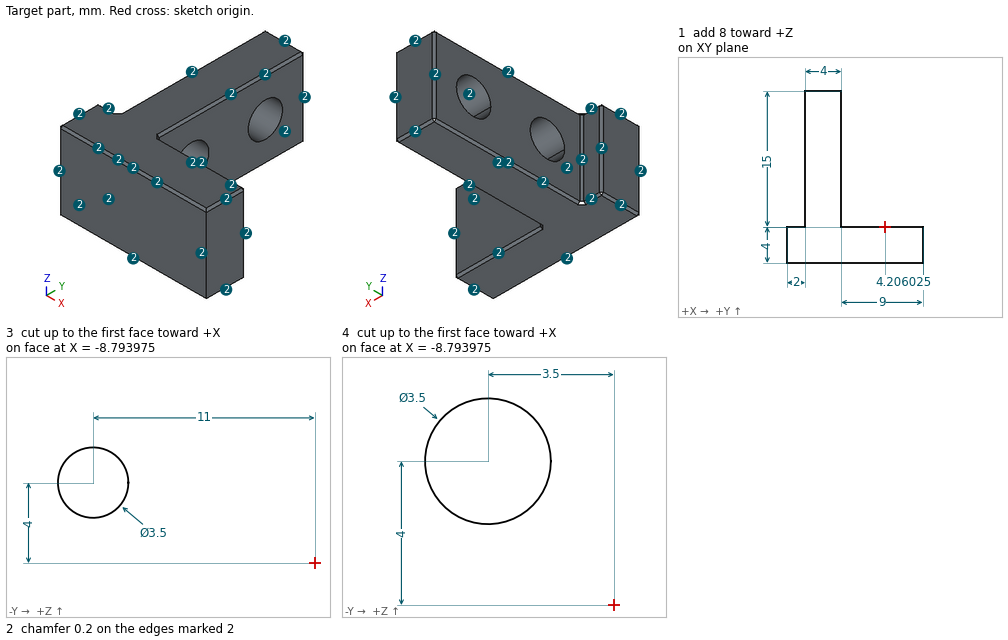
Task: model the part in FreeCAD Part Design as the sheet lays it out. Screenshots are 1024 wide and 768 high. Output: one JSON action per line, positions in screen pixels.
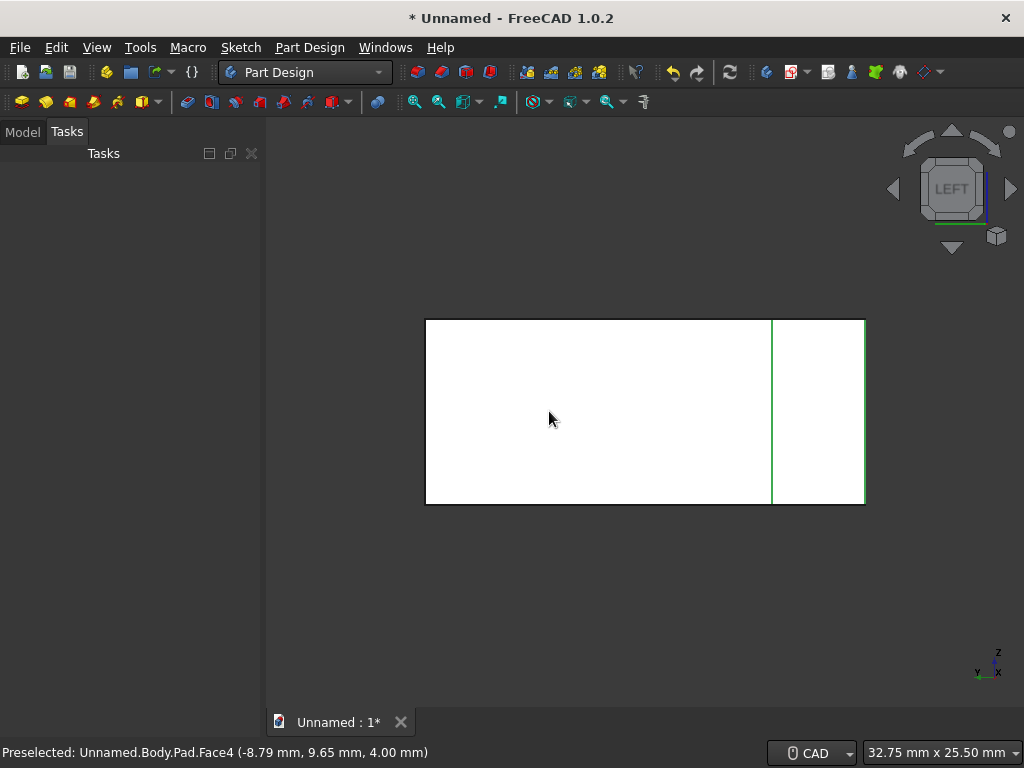
{"action": "left_click", "coordinate": [442, 72]}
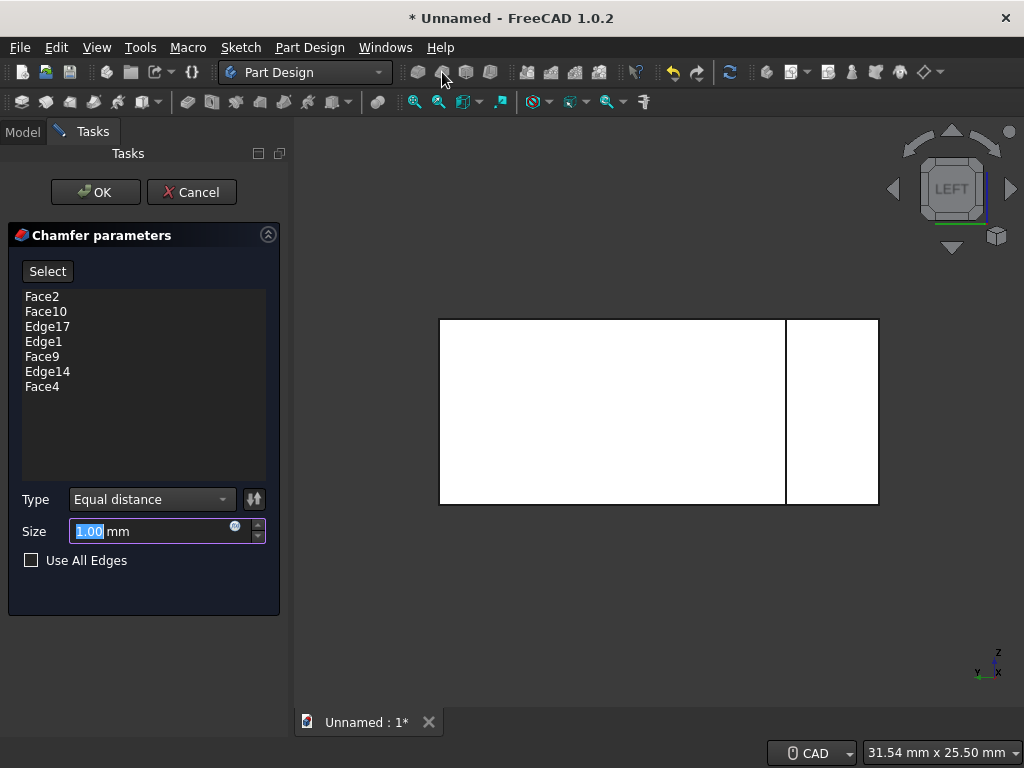
{"action": "type", "text": "0.2"}
{"action": "key", "text": "Tab"}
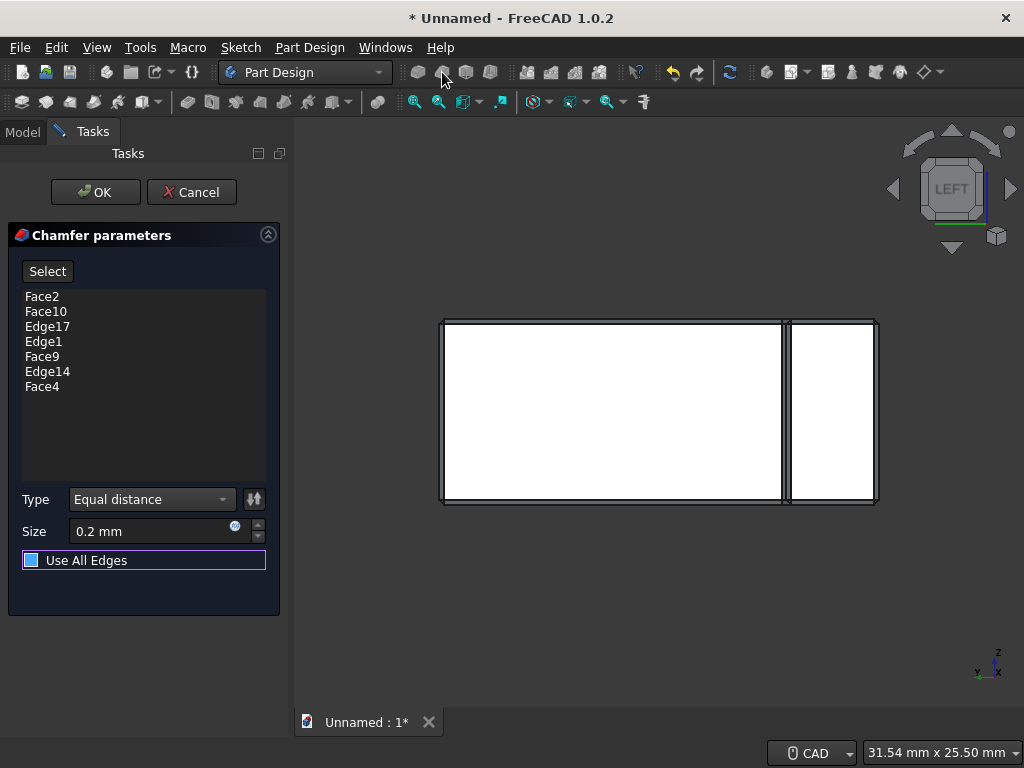
{"action": "left_click", "coordinate": [96, 192]}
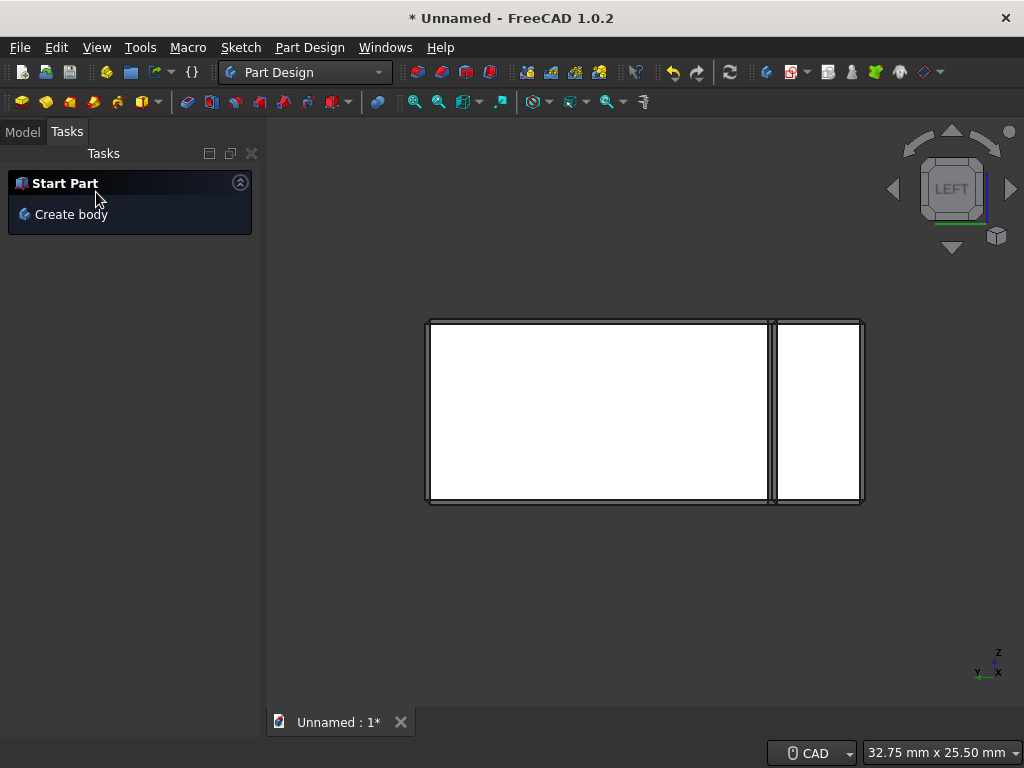
{"action": "left_click", "coordinate": [550, 411]}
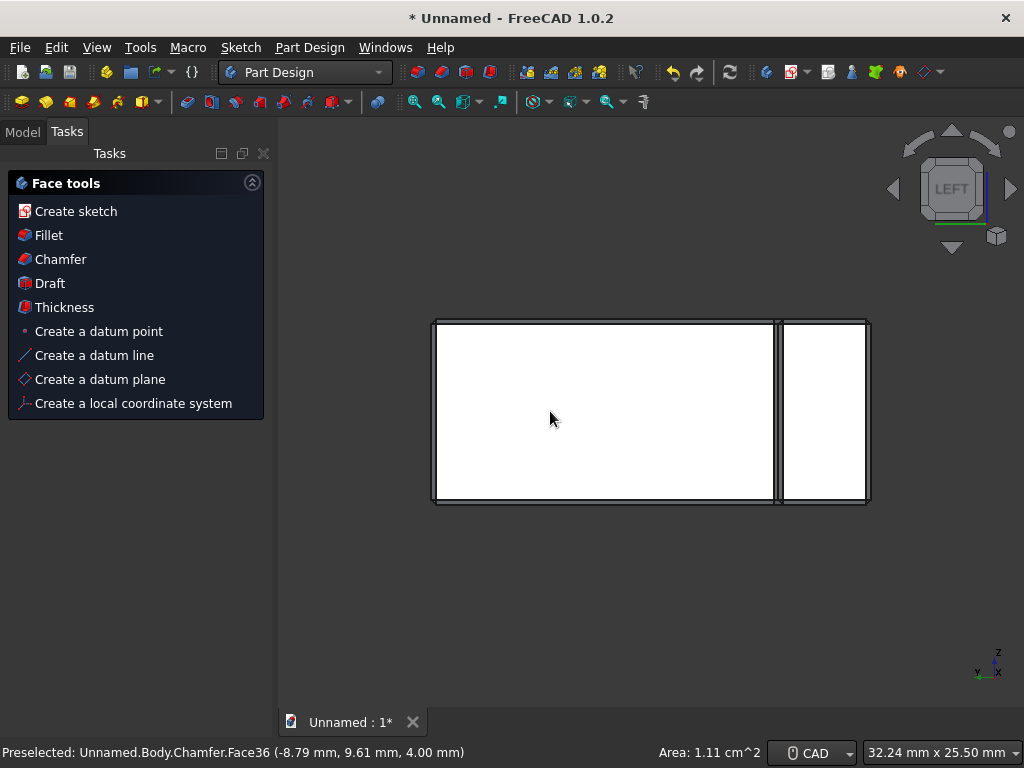
{"action": "left_click", "coordinate": [792, 72]}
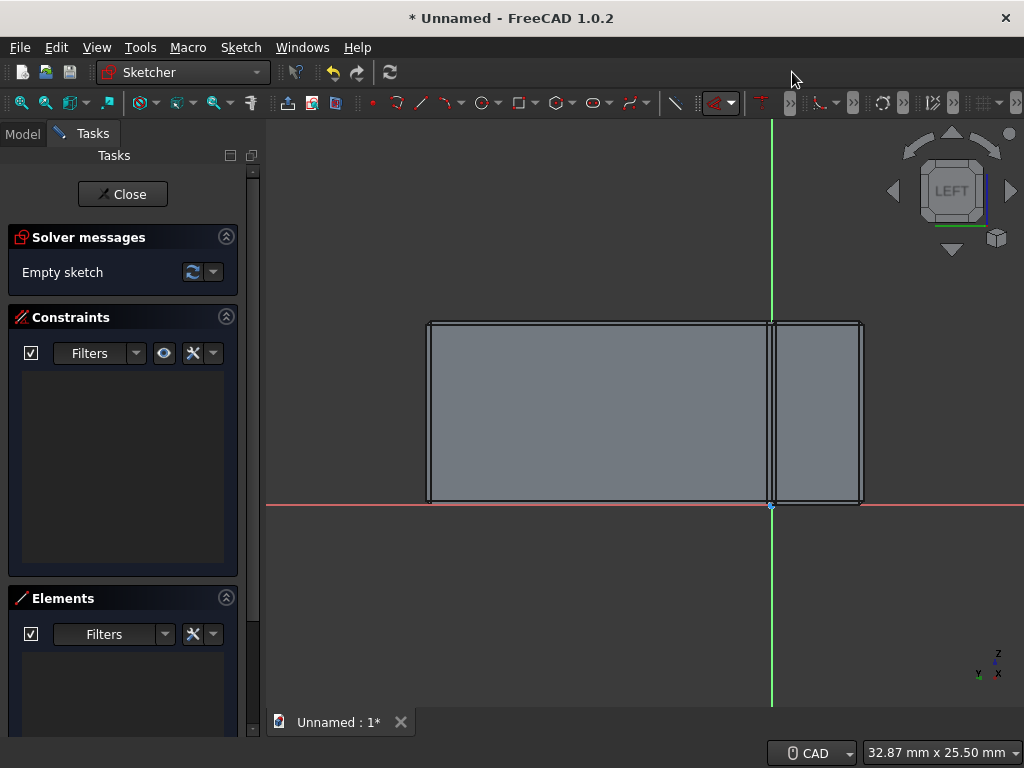
{"action": "left_click", "coordinate": [336, 104]}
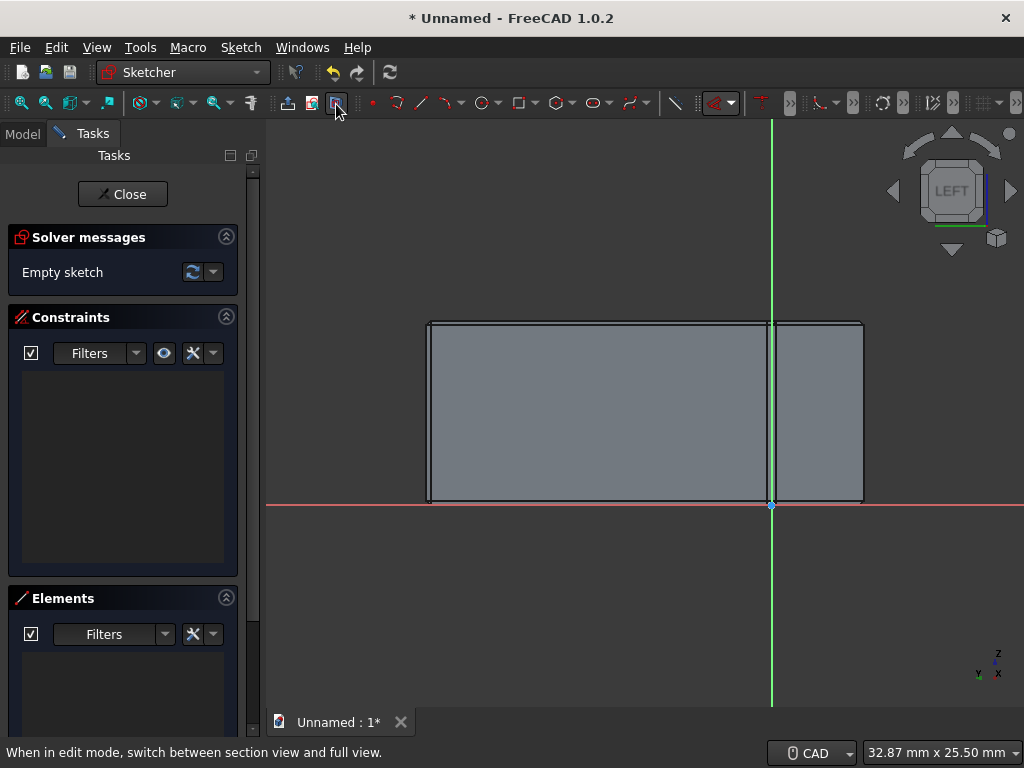
{"action": "scroll", "coordinate": [503, 413], "scroll_direction": "up", "scroll_amount": 8}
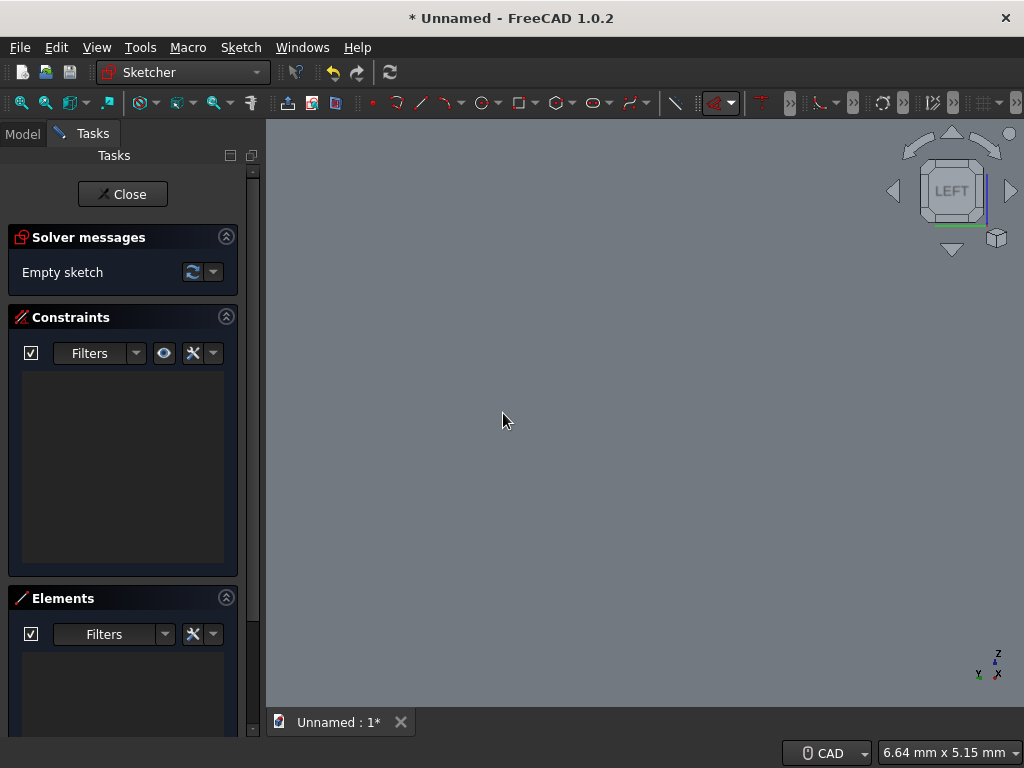
{"action": "left_click", "coordinate": [482, 104]}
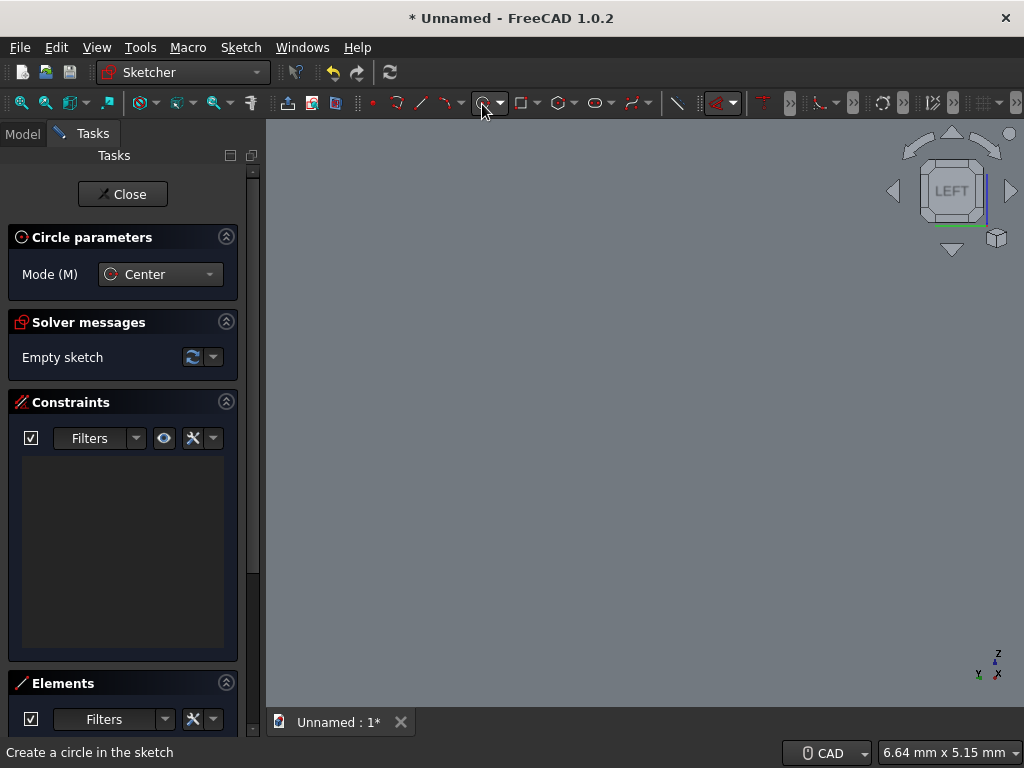
{"action": "left_click", "coordinate": [577, 411]}
{"action": "left_click", "coordinate": [718, 270]}
{"action": "key", "text": "Escape"}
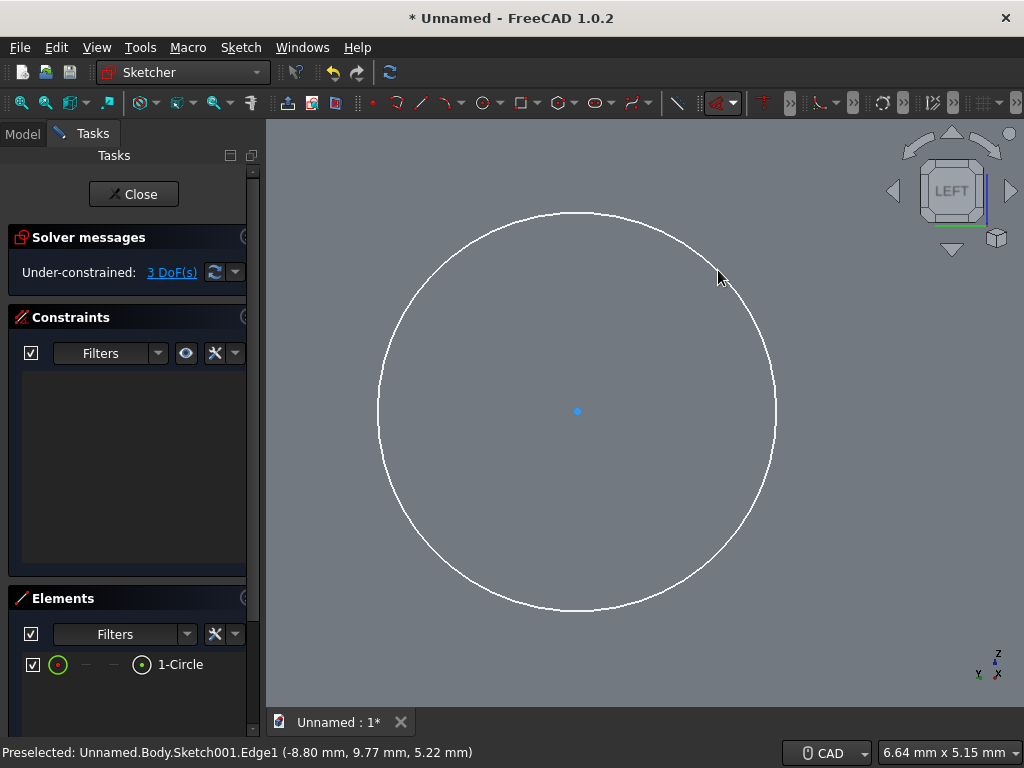
{"action": "left_click", "coordinate": [718, 271]}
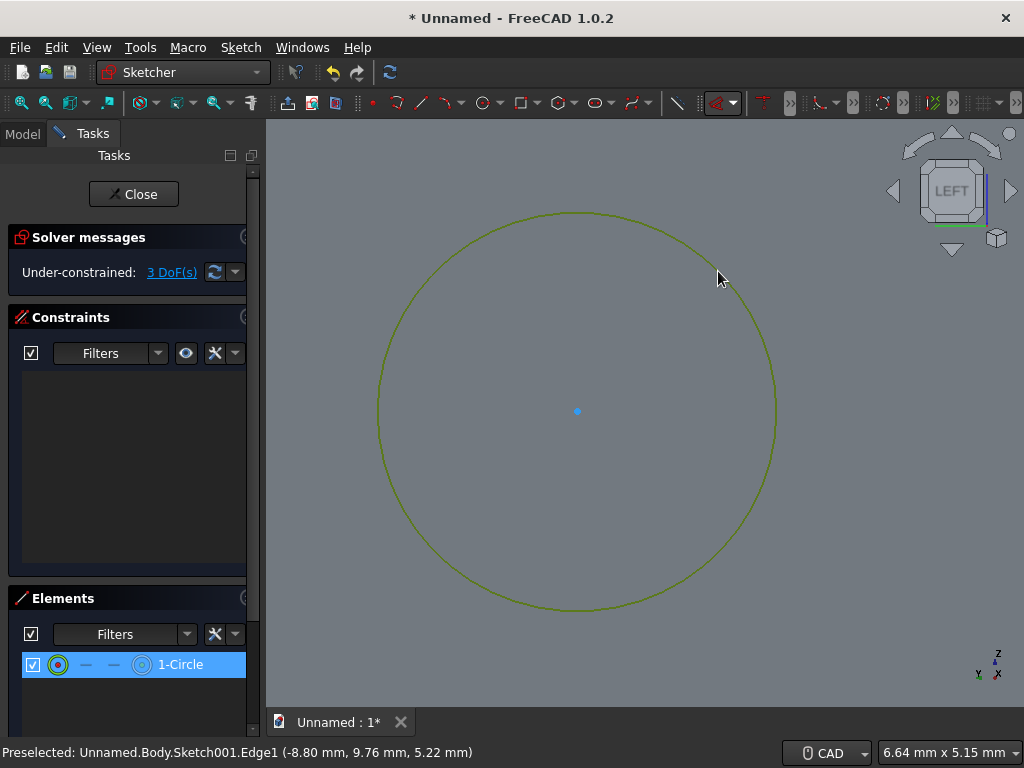
{"action": "key", "text": "k o"}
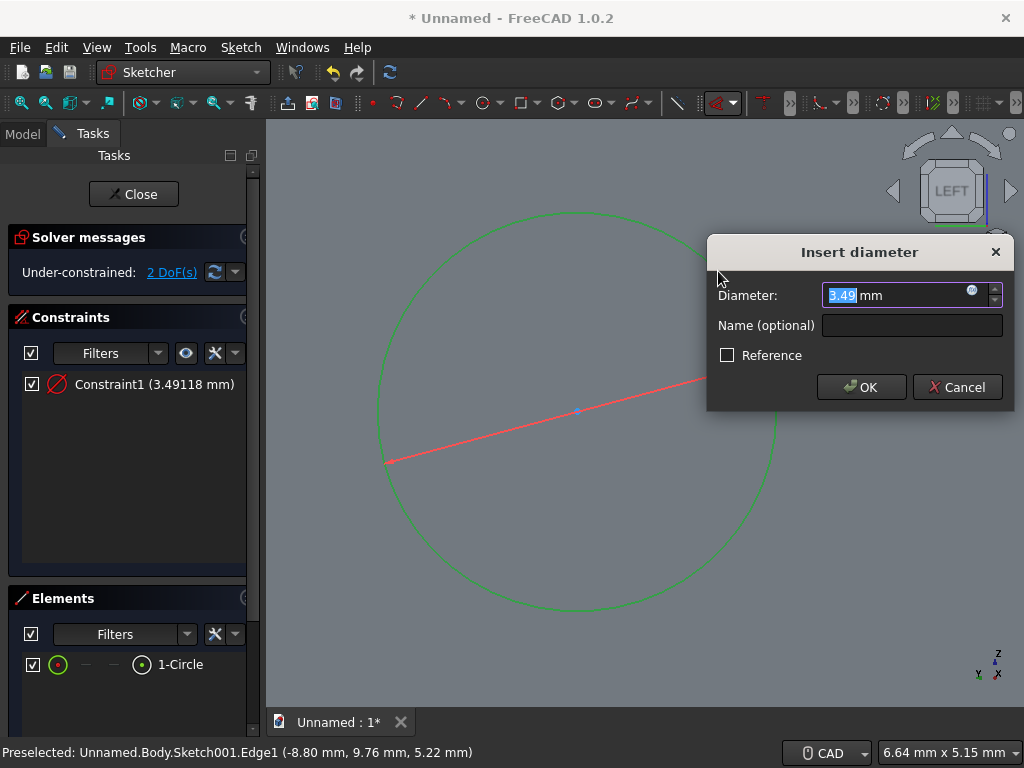
{"action": "type", "text": "3.5"}
{"action": "key", "text": "Return"}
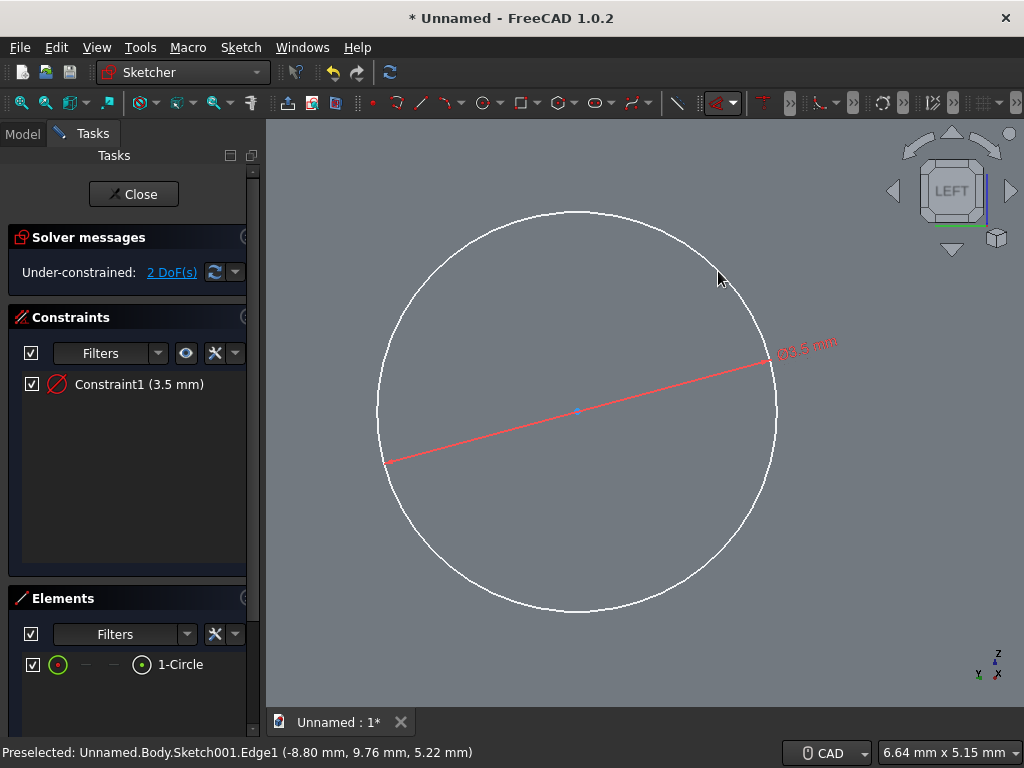
{"action": "left_click", "coordinate": [577, 412]}